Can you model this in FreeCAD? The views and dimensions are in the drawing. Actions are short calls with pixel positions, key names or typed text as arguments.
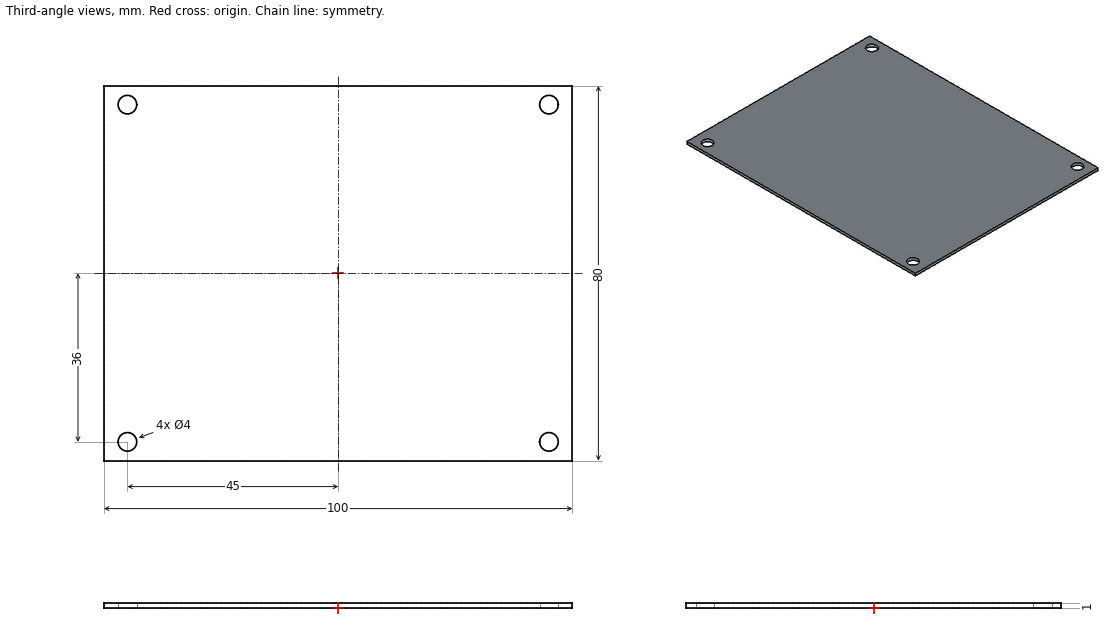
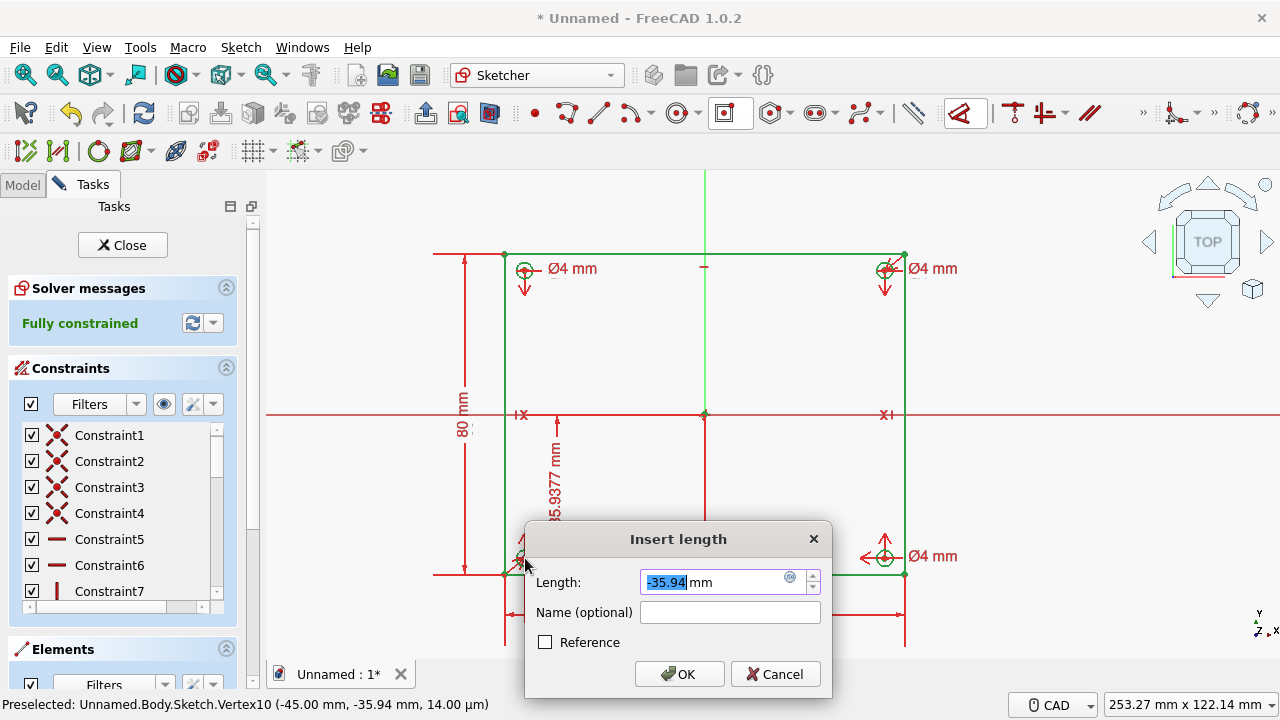
text(-36)
key(Return)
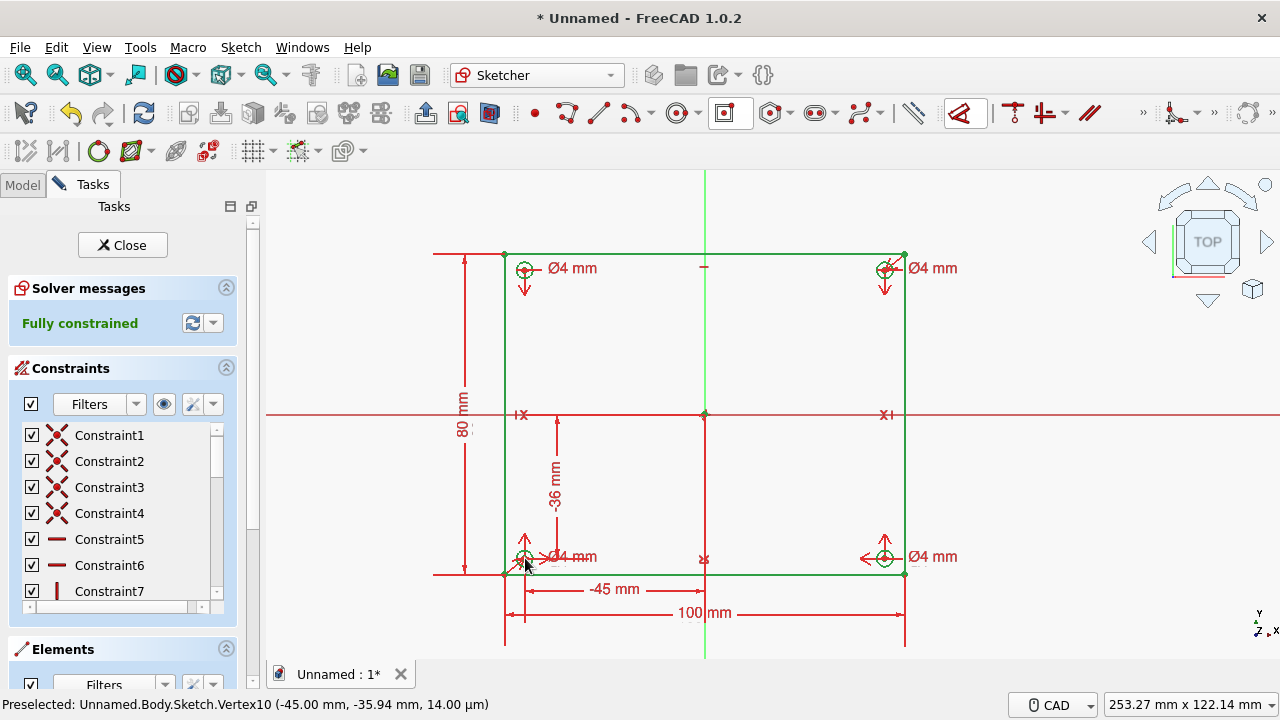
click(123, 245)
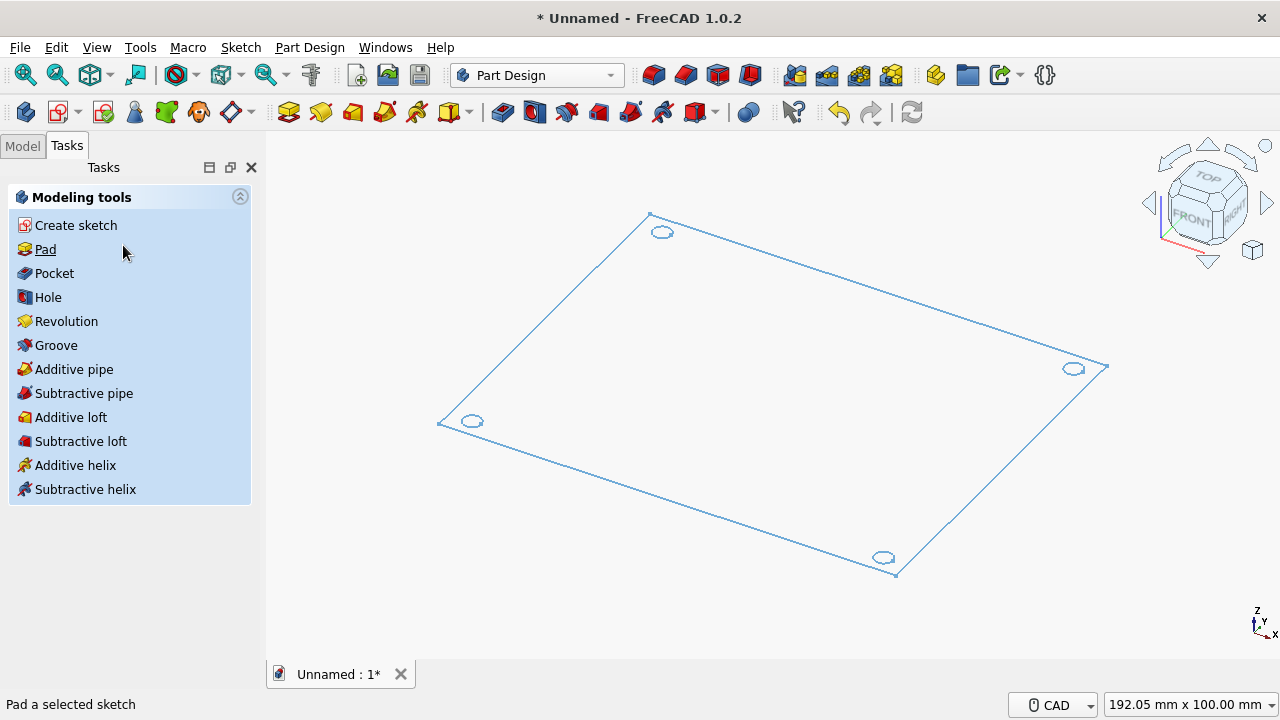
click(290, 112)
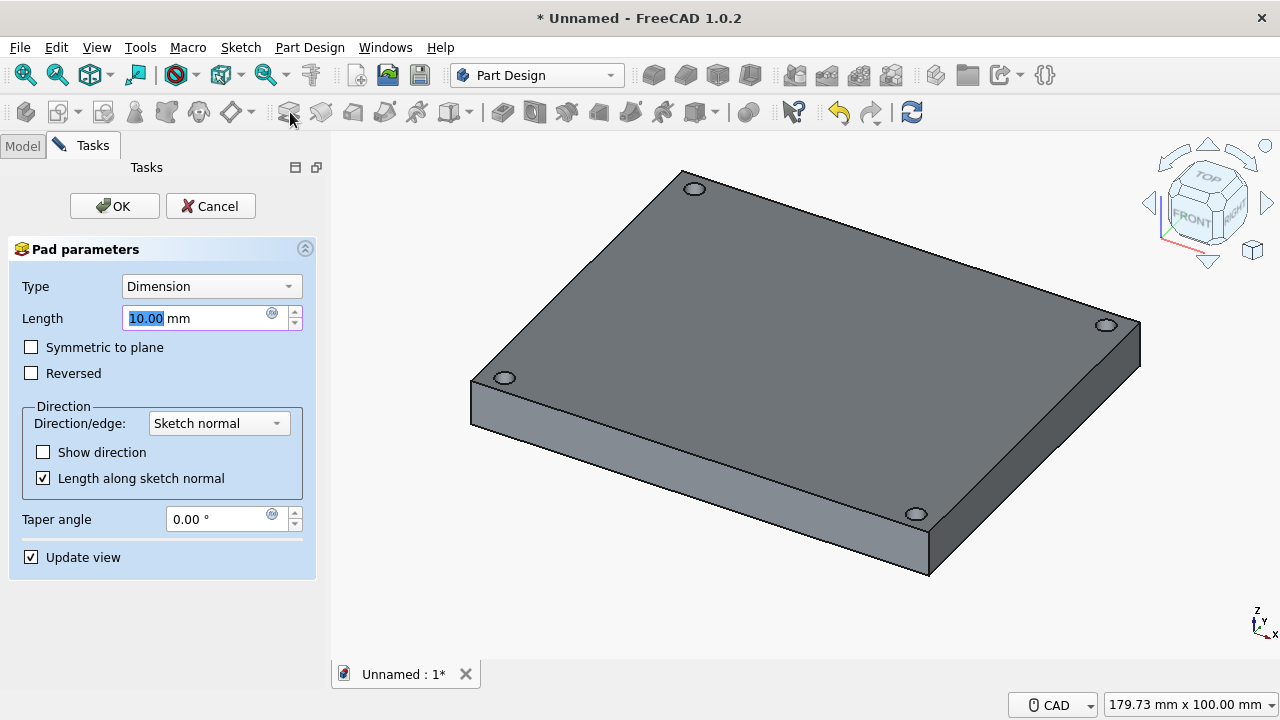
text(1)
key(Tab)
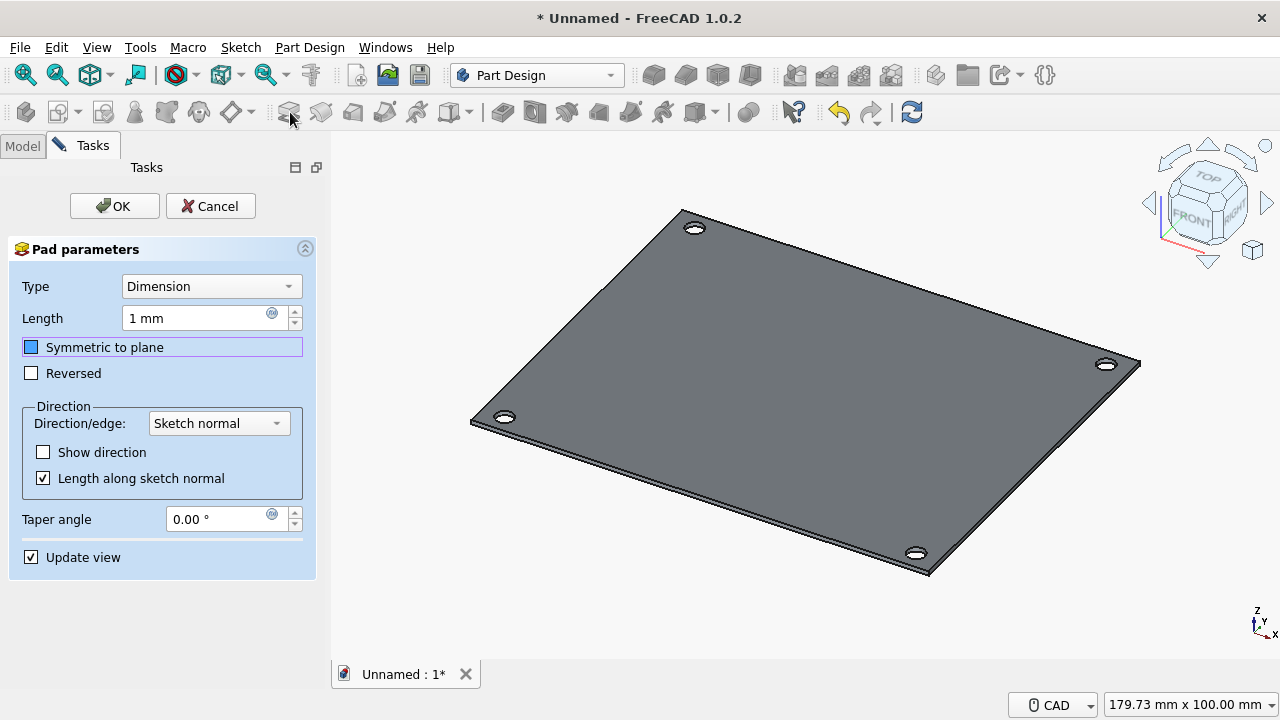
click(115, 206)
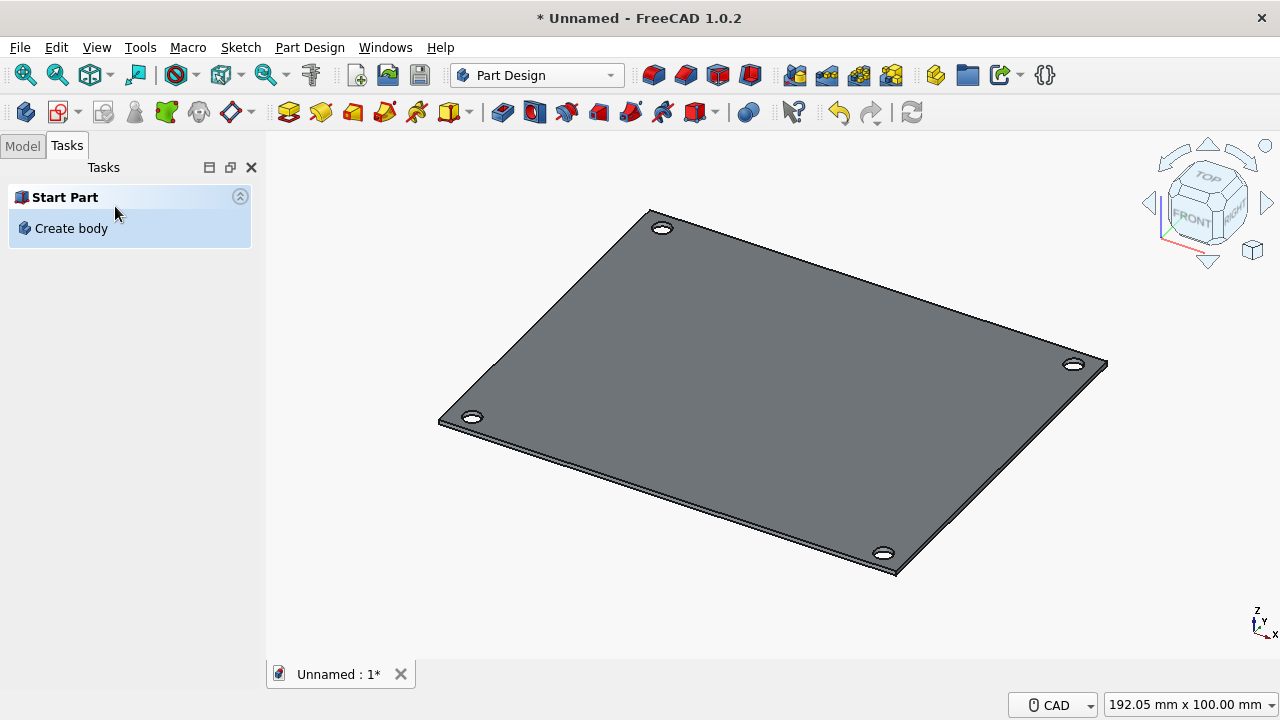
key(0)